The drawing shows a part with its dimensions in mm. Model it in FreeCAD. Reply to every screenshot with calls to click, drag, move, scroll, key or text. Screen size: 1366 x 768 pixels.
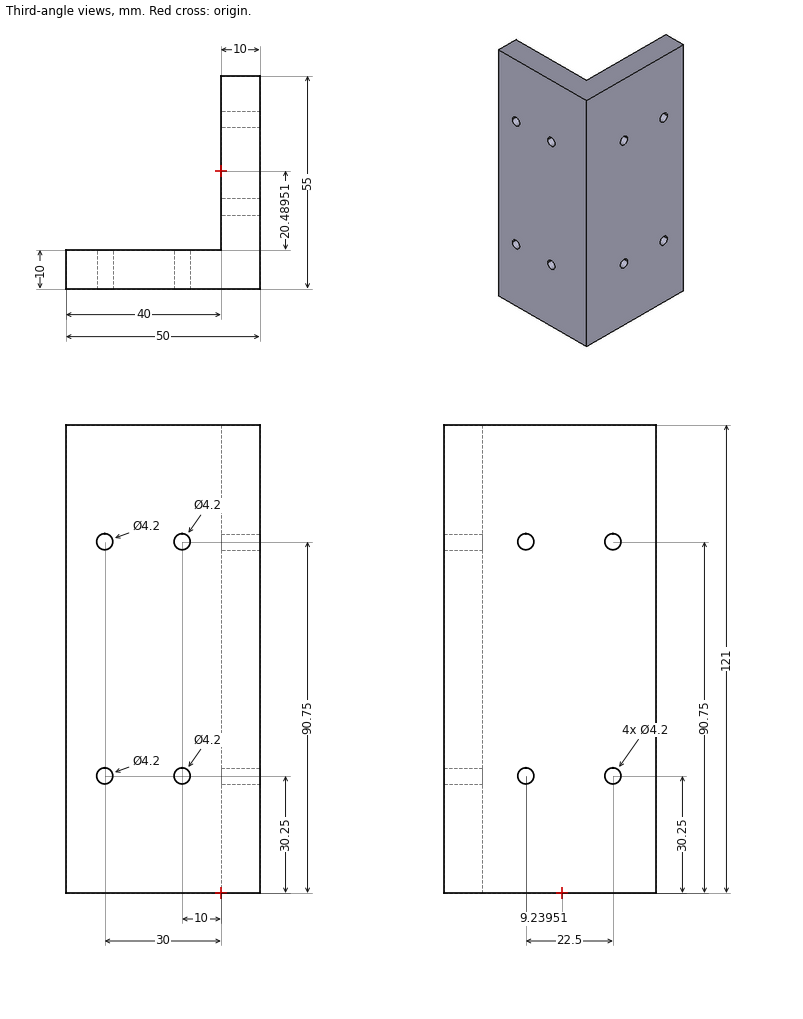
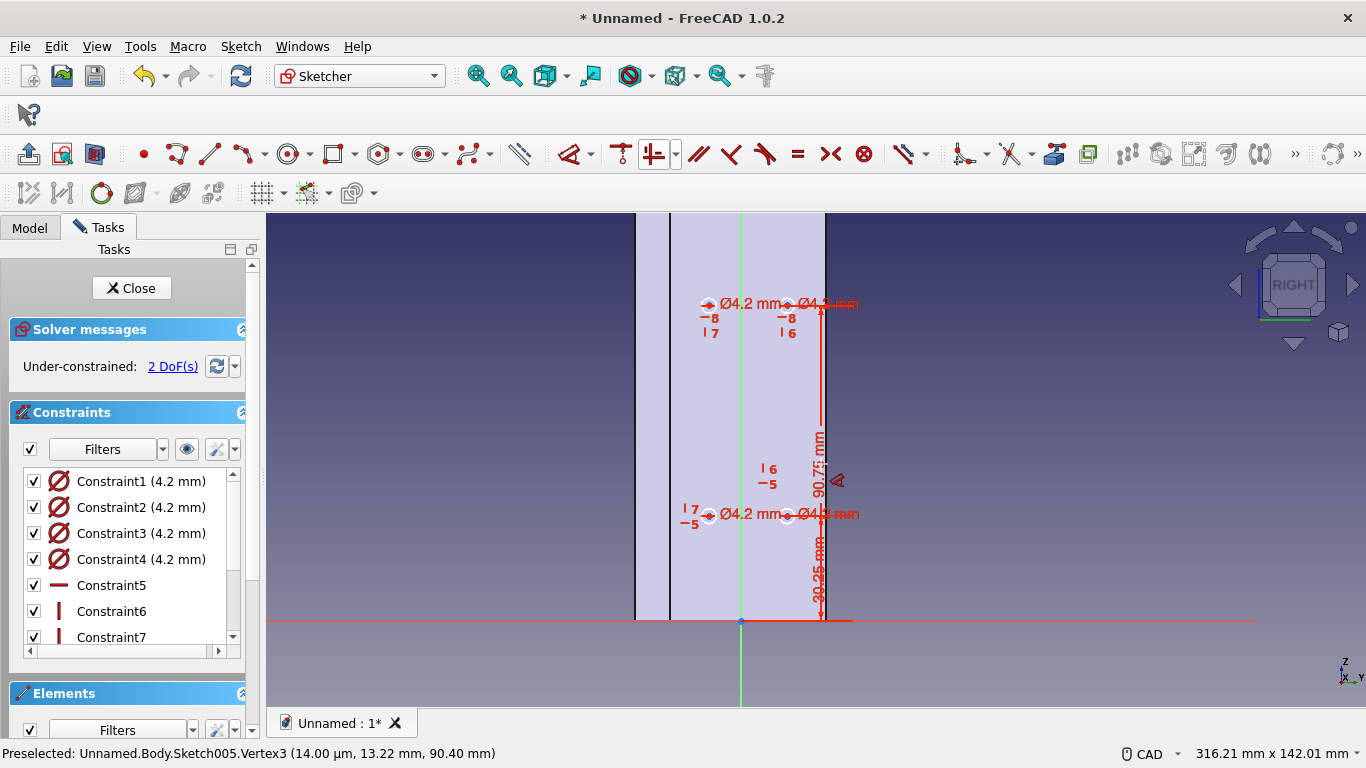
click(787, 516)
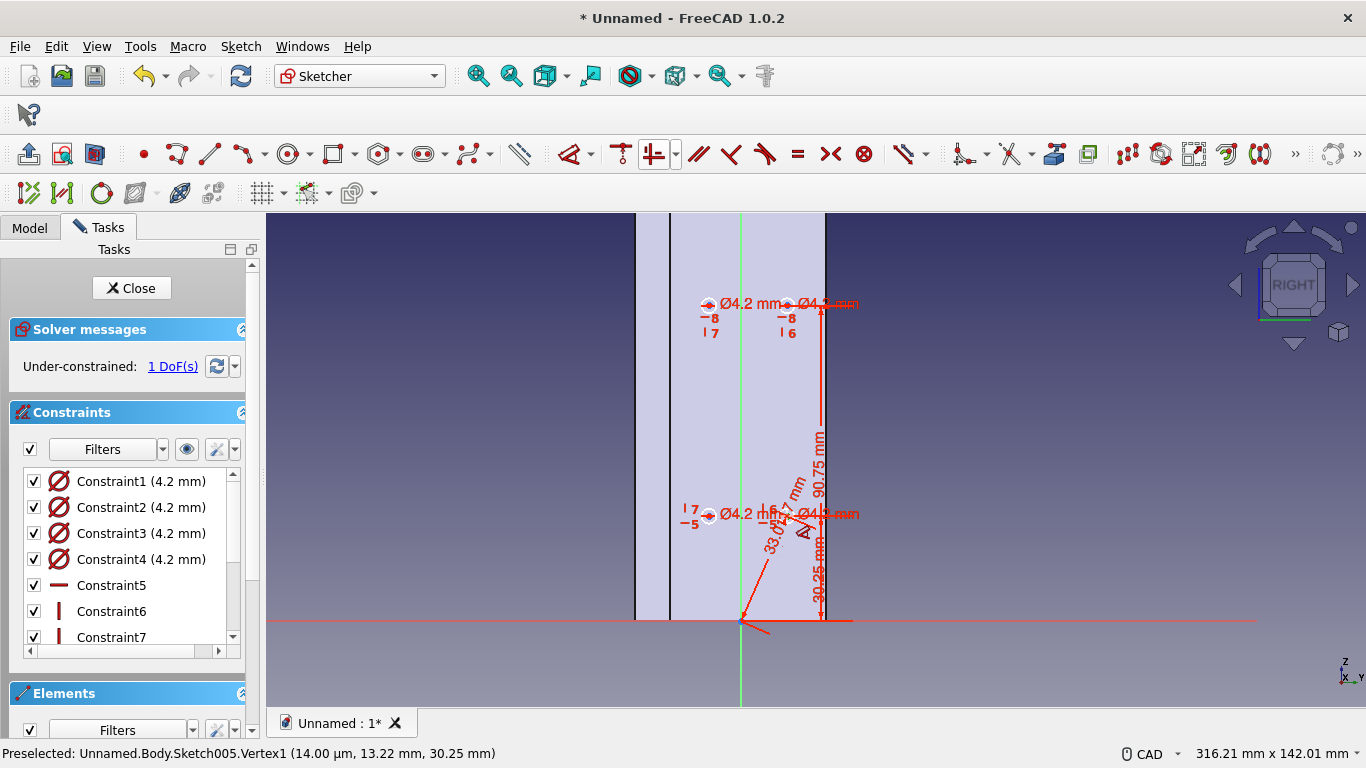
click(709, 516)
click(721, 550)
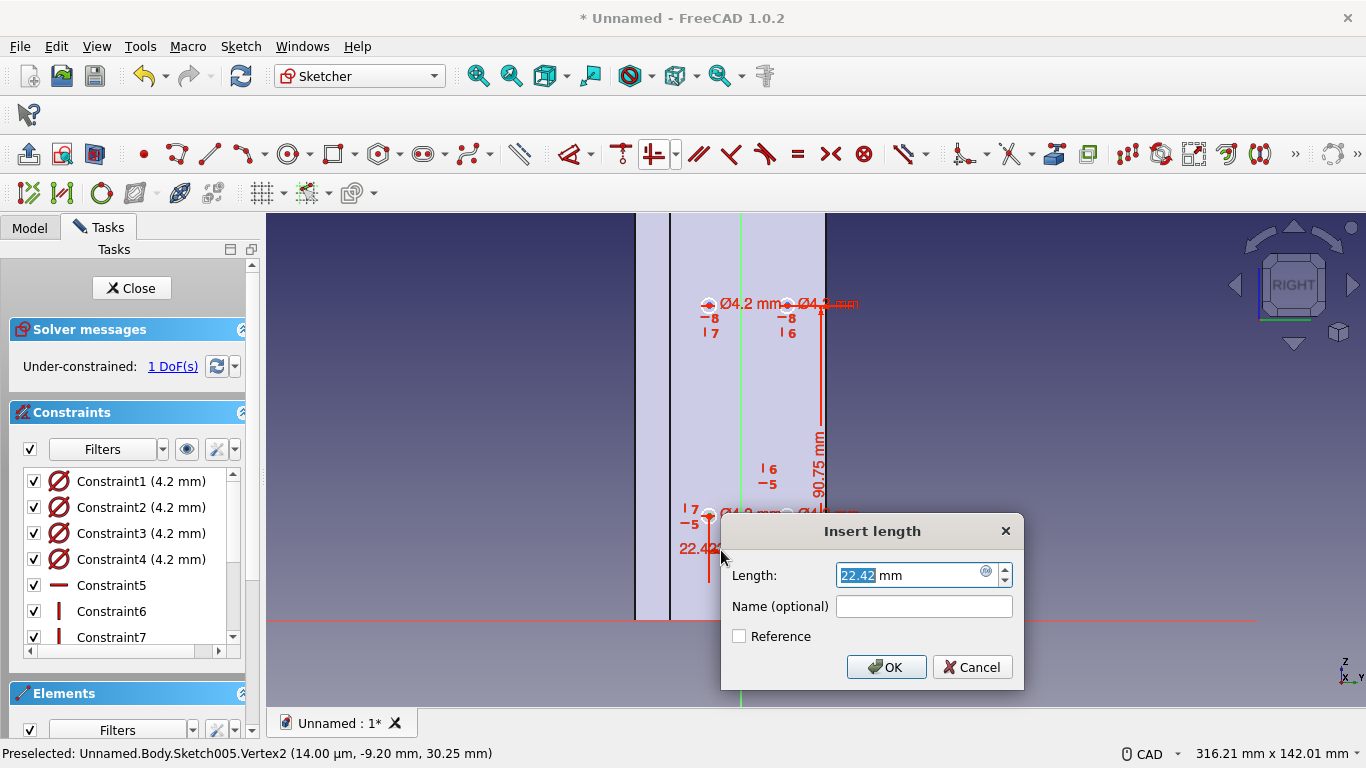
text(22.5)
key(Return)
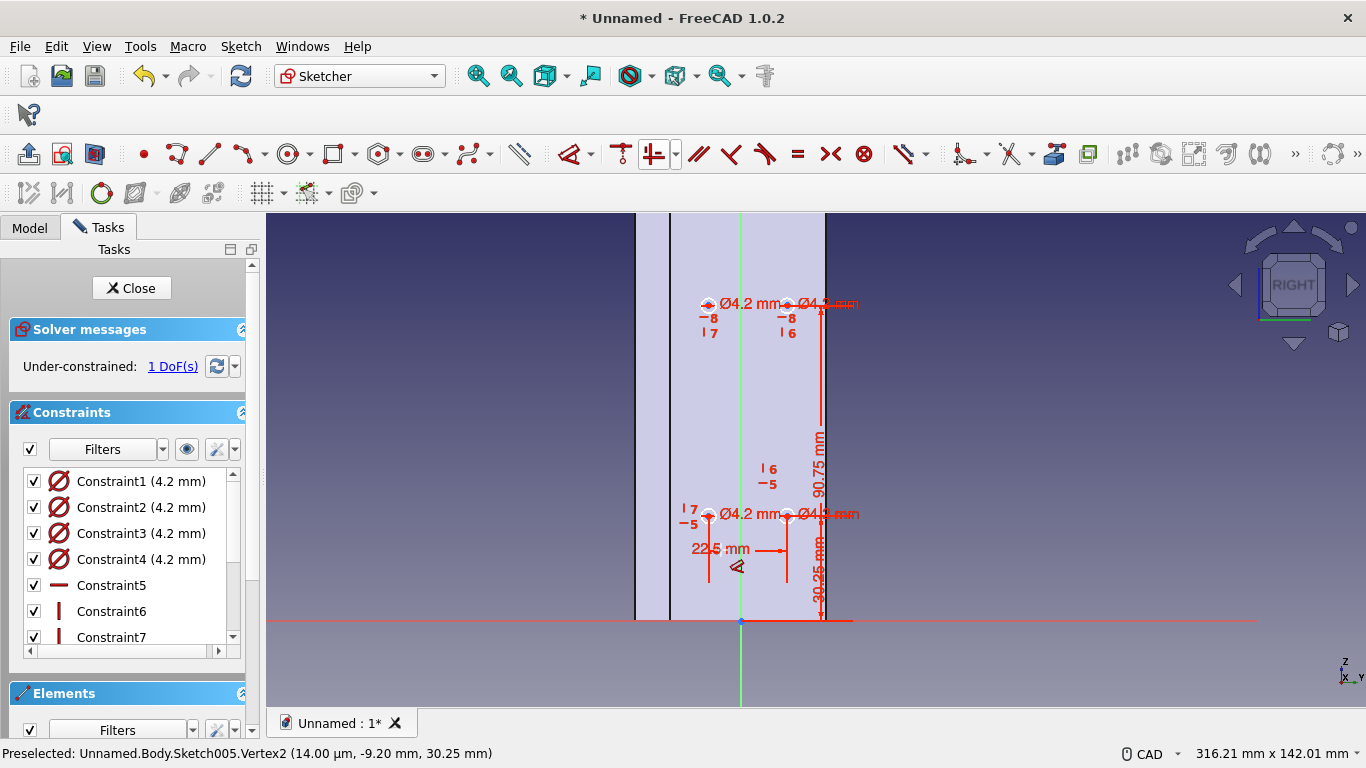
scroll(709, 516, up, 2)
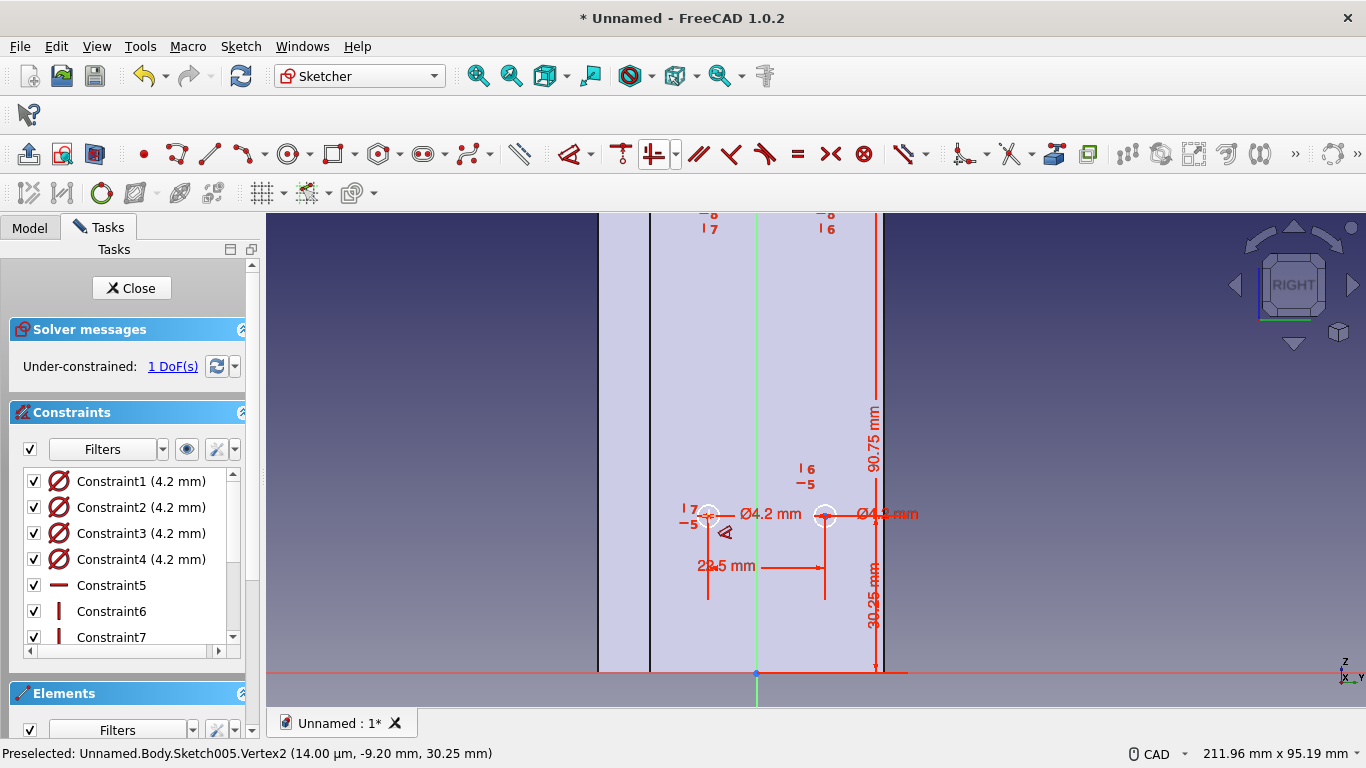
click(708, 516)
click(732, 482)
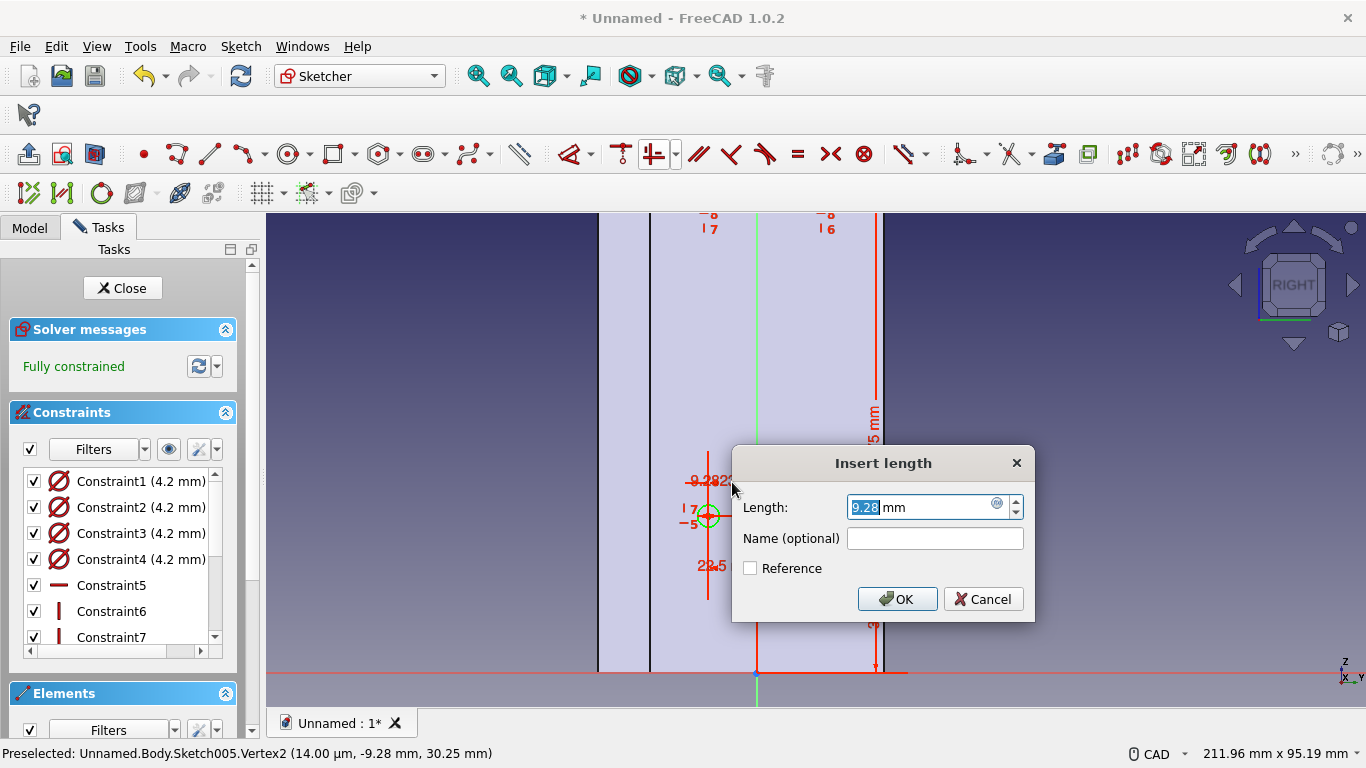
text(9.23951)
key(Return)
key(Escape)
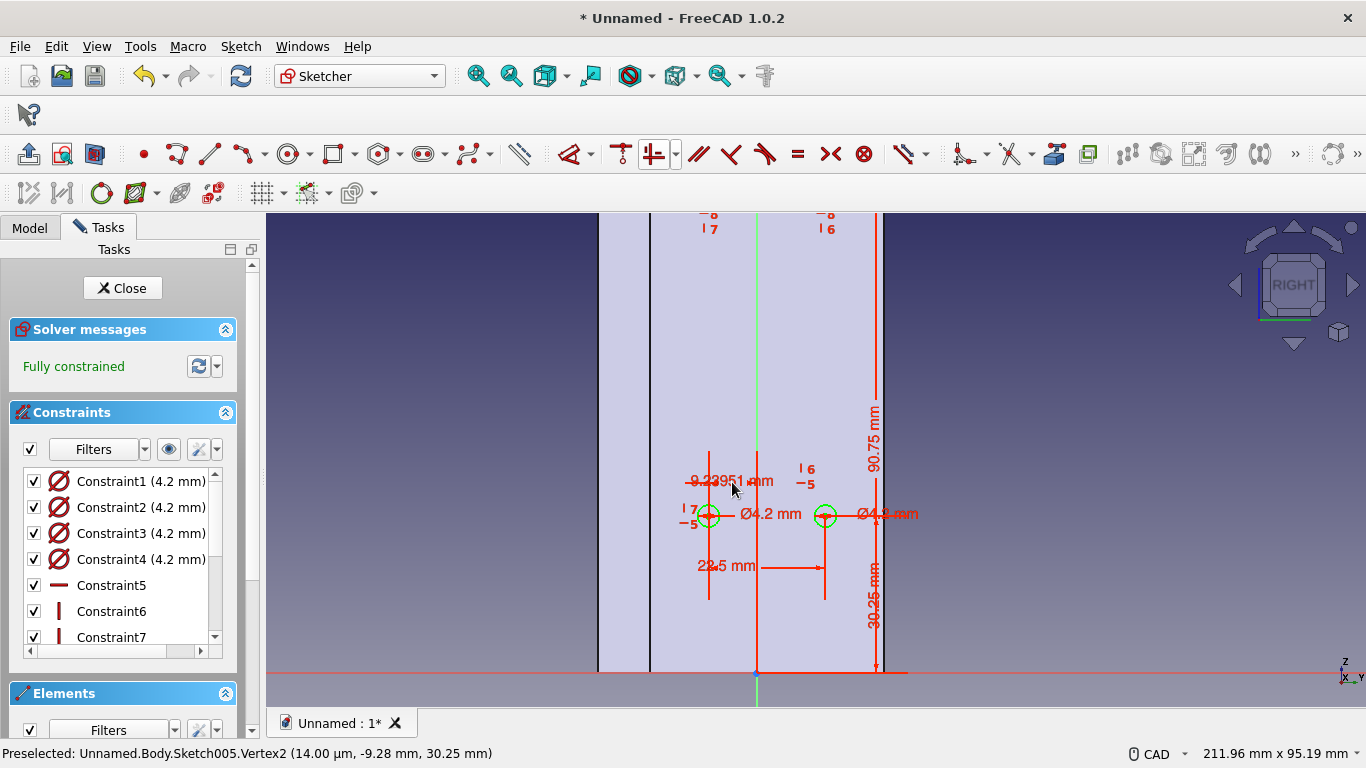
click(123, 288)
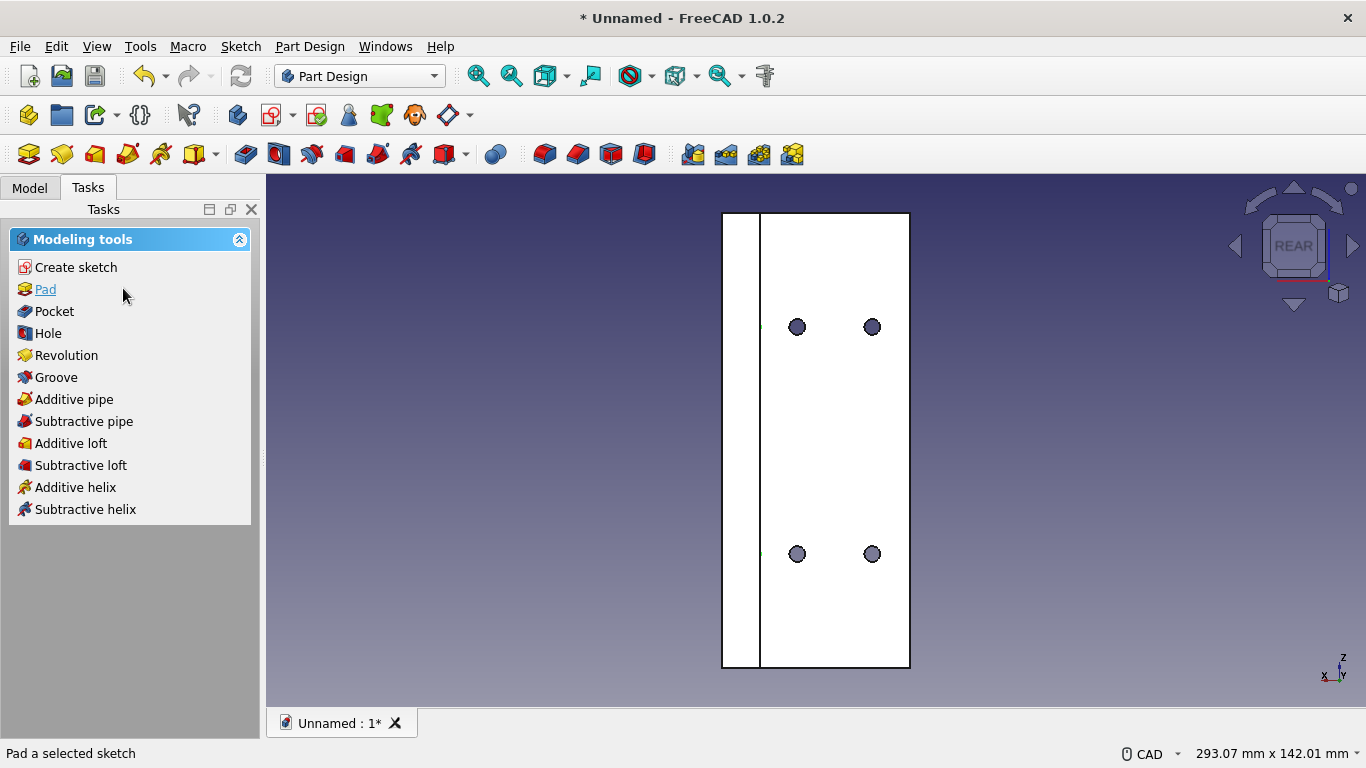
click(246, 154)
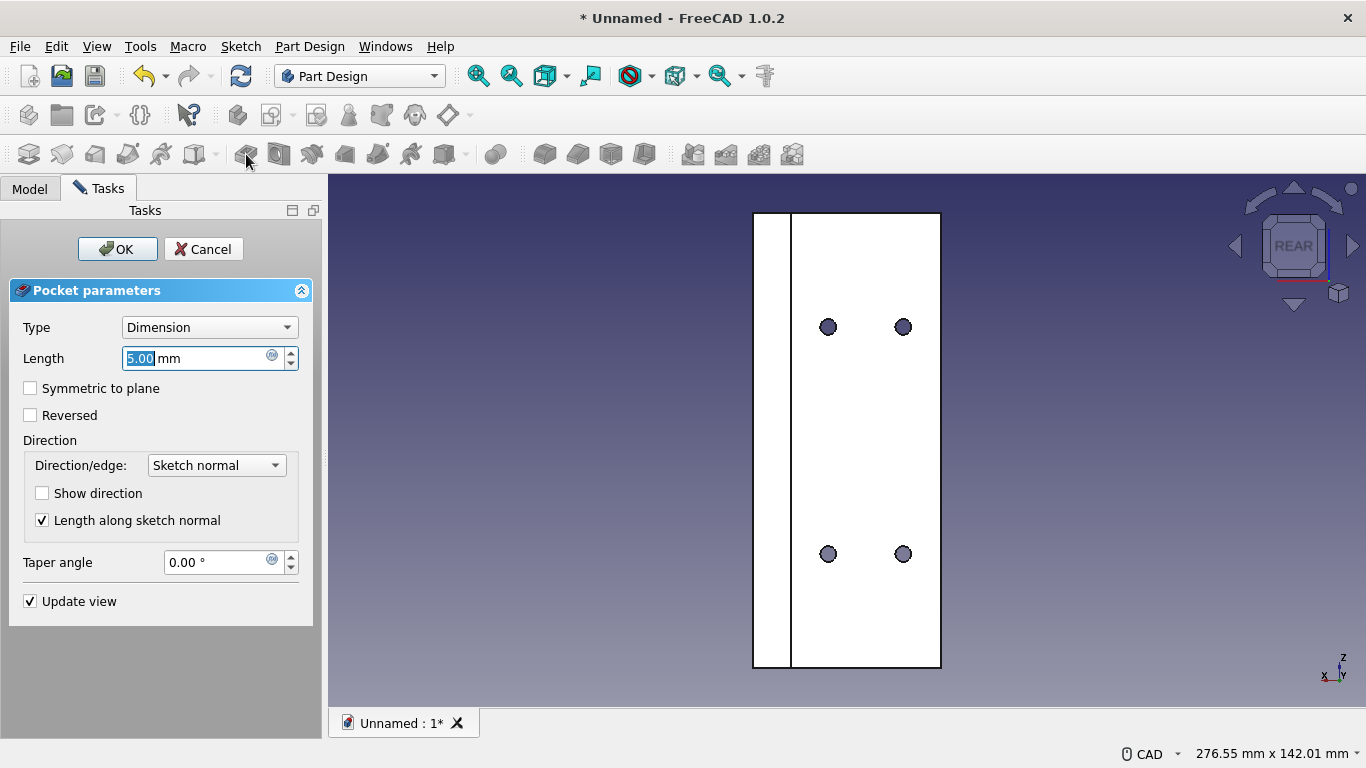
text(10)
key(Tab)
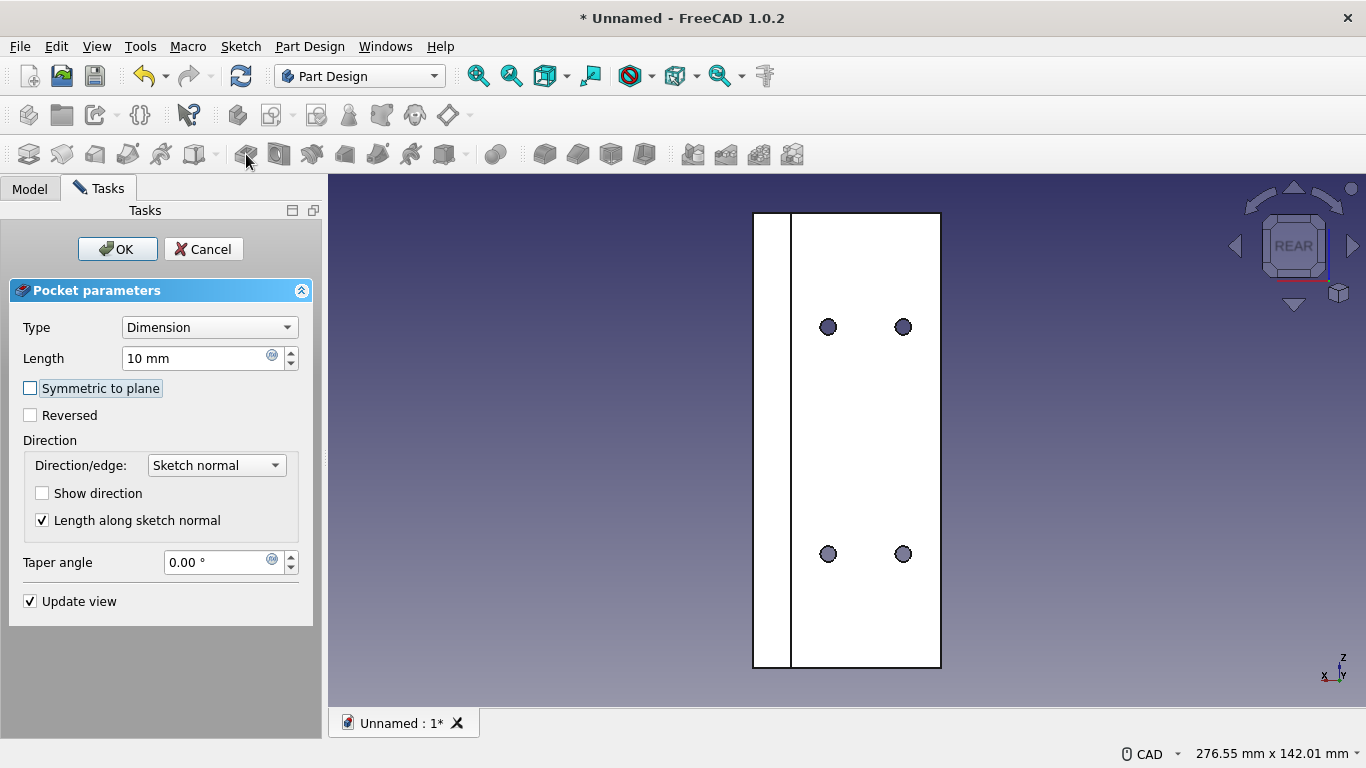
click(31, 415)